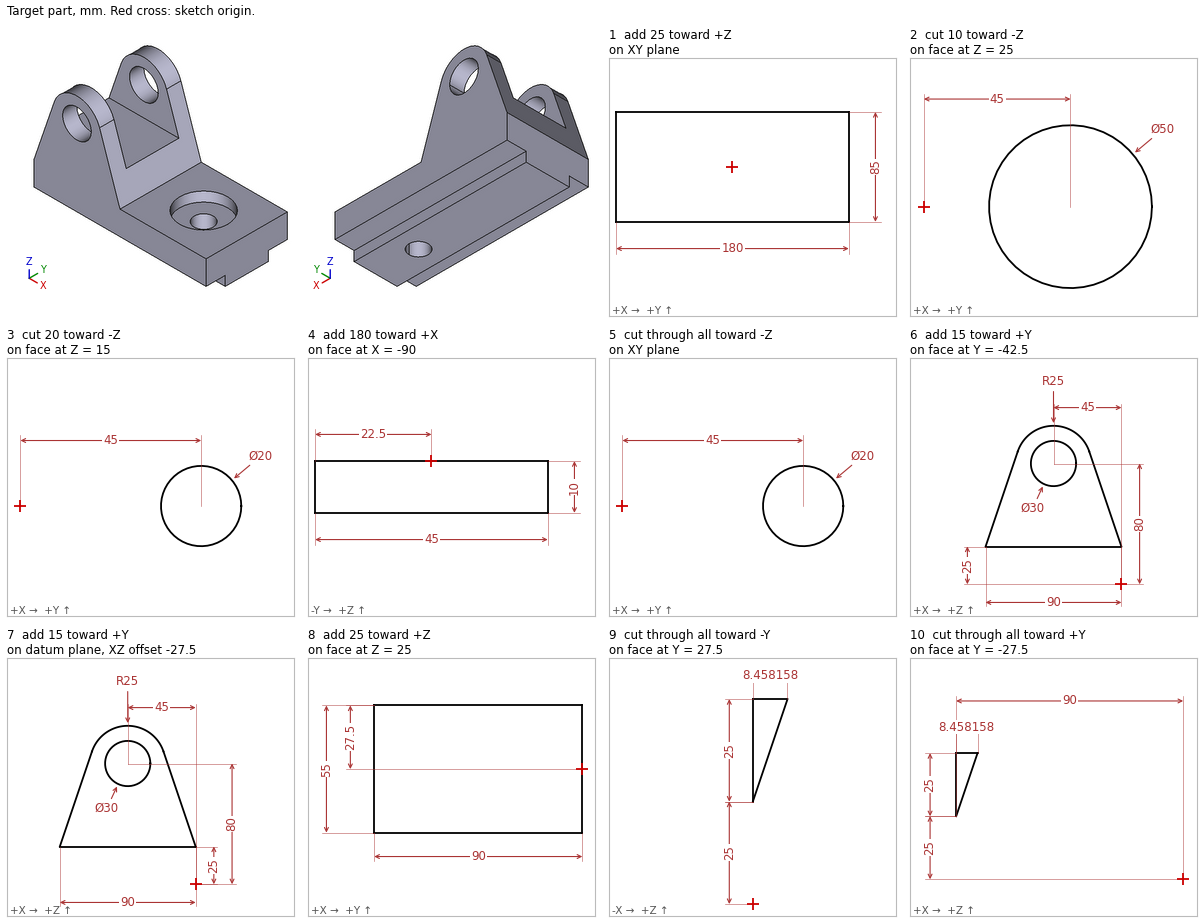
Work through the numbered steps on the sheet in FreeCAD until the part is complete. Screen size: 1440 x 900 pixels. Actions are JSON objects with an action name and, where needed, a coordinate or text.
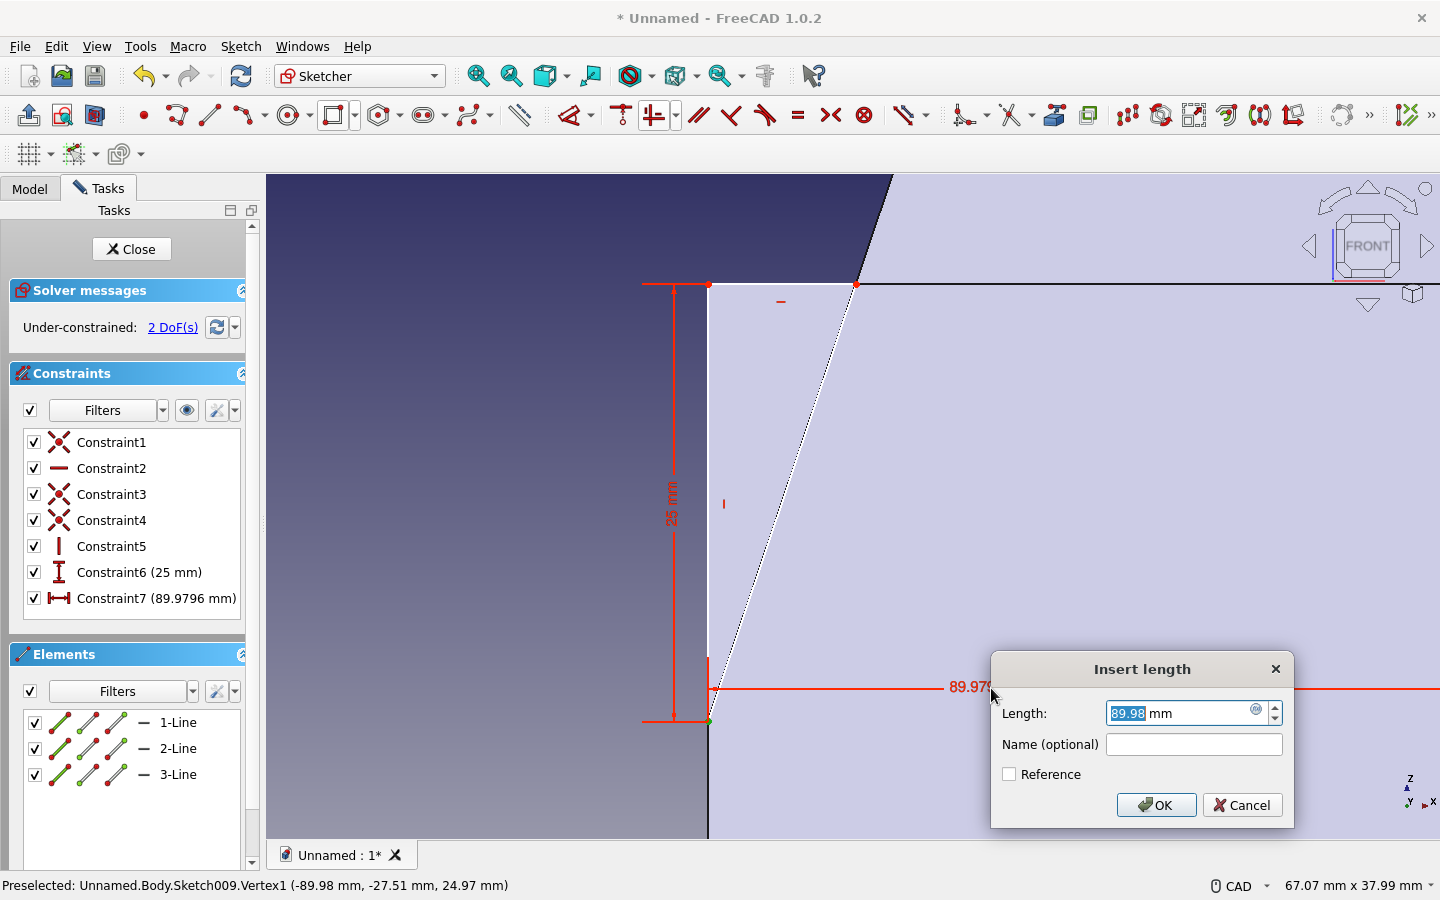
{"action": "type", "text": "90"}
{"action": "key", "text": "Return"}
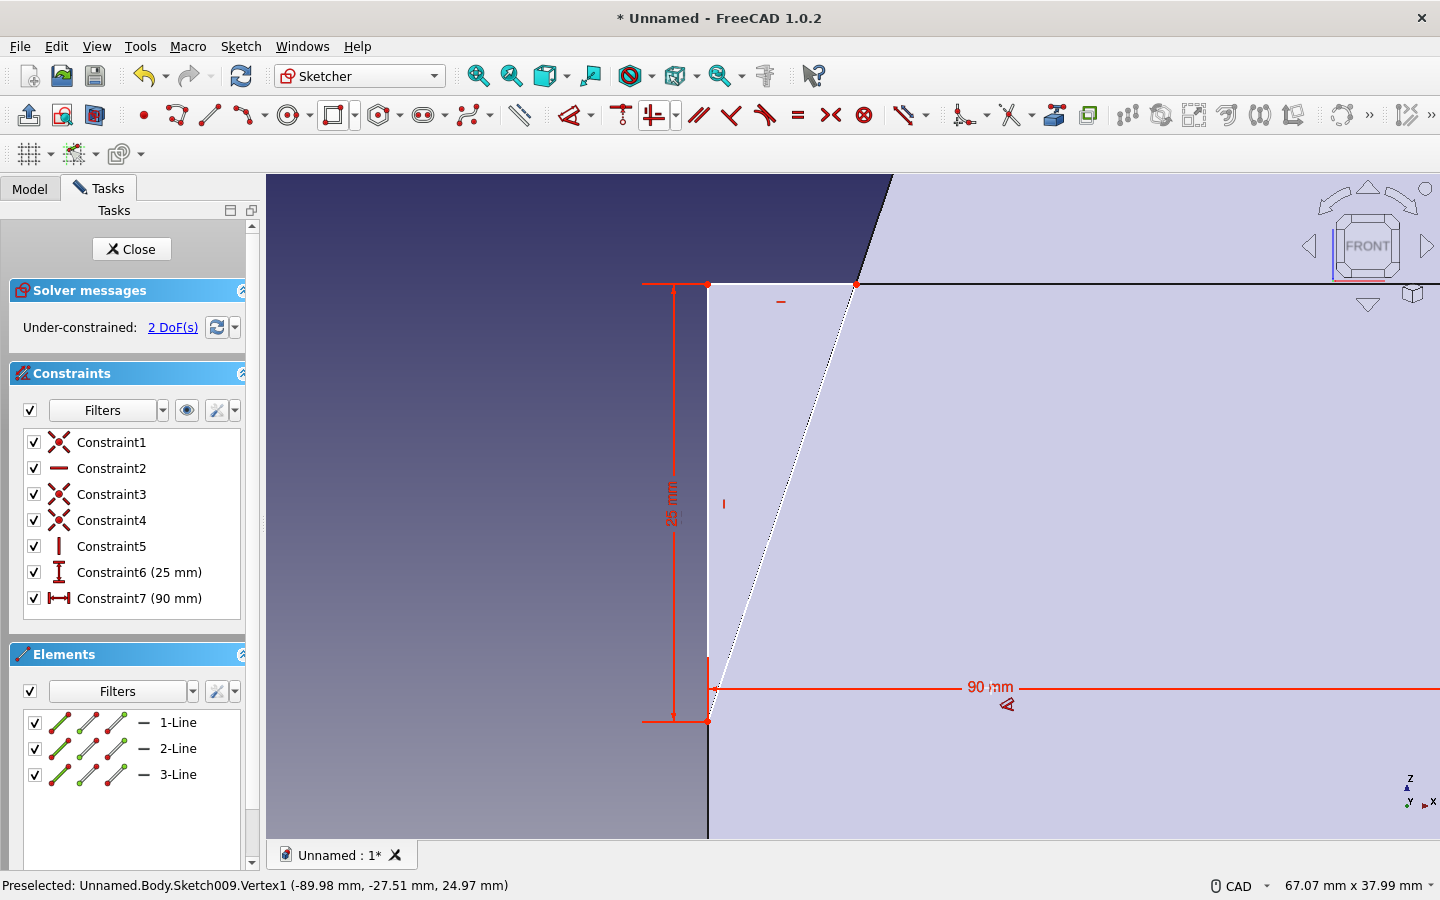
{"action": "left_click", "coordinate": [708, 722]}
{"action": "left_click", "coordinate": [674, 767]}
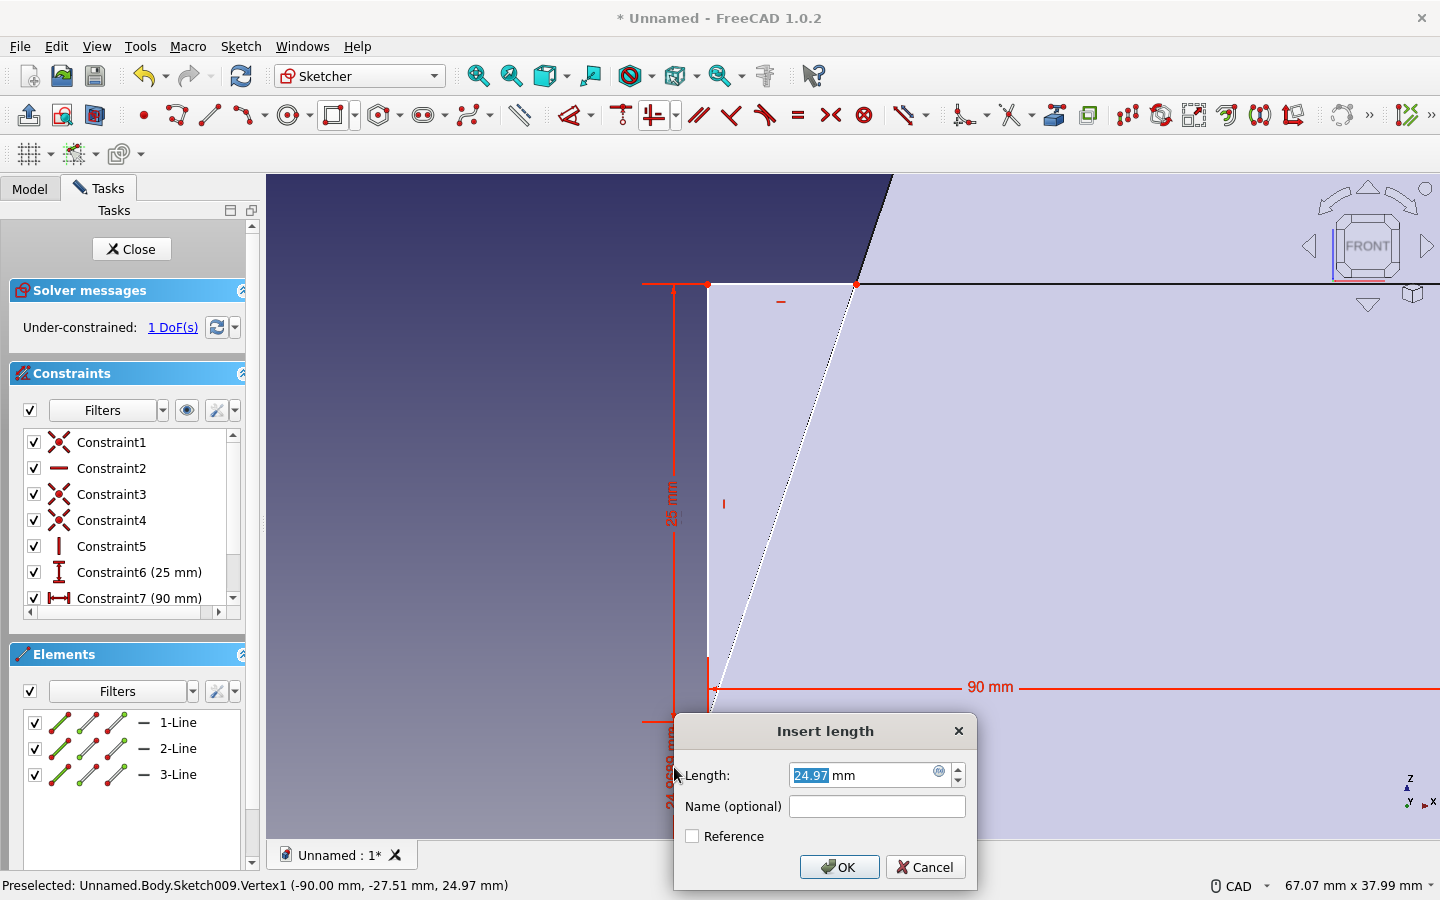
{"action": "type", "text": "25"}
{"action": "key", "text": "Return"}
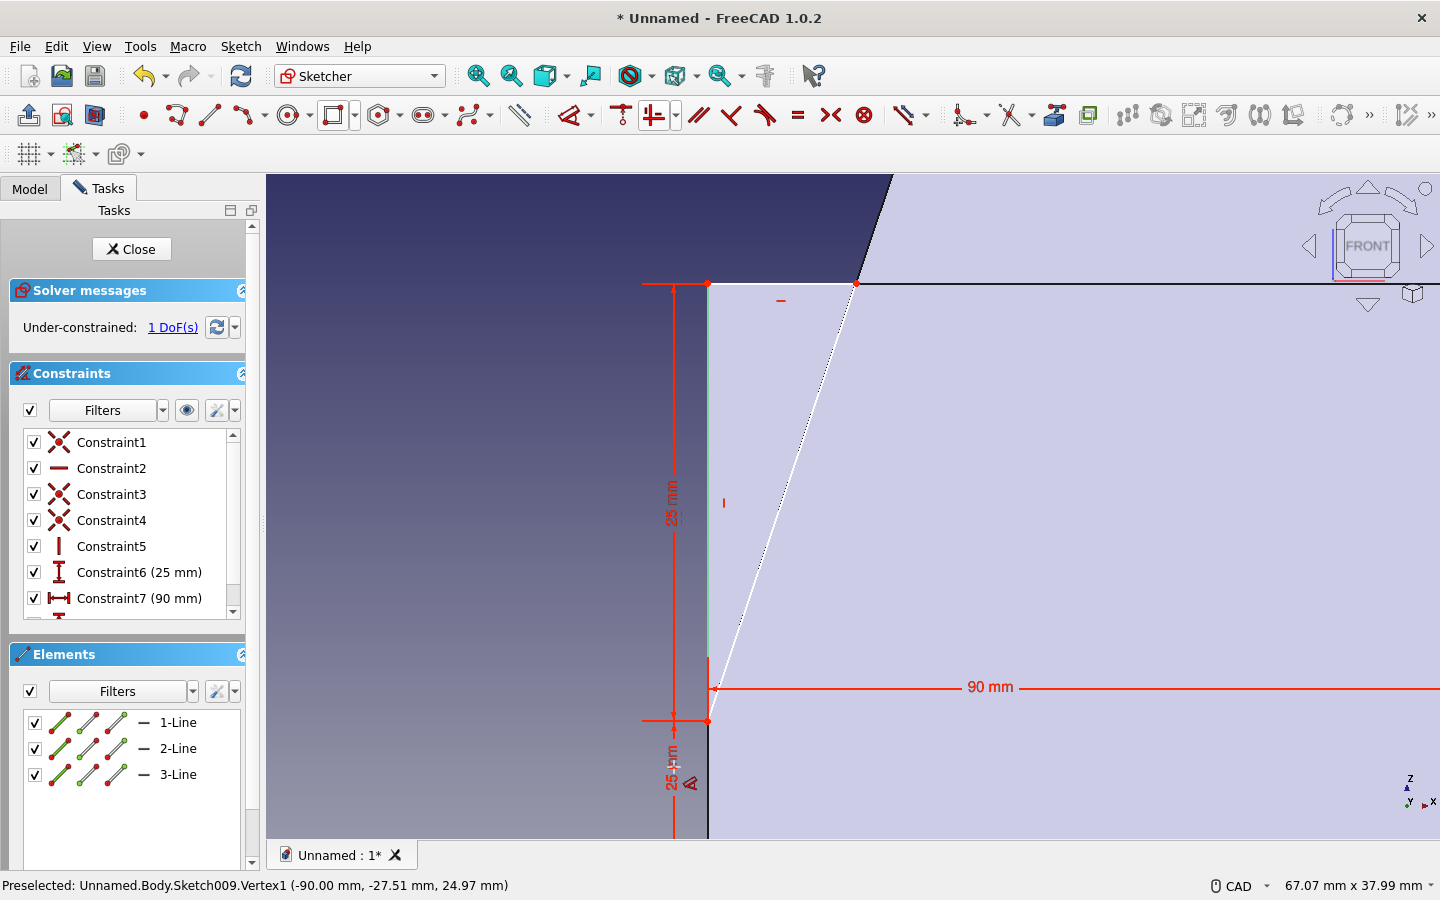
{"action": "left_click", "coordinate": [811, 284]}
{"action": "left_click", "coordinate": [782, 250]}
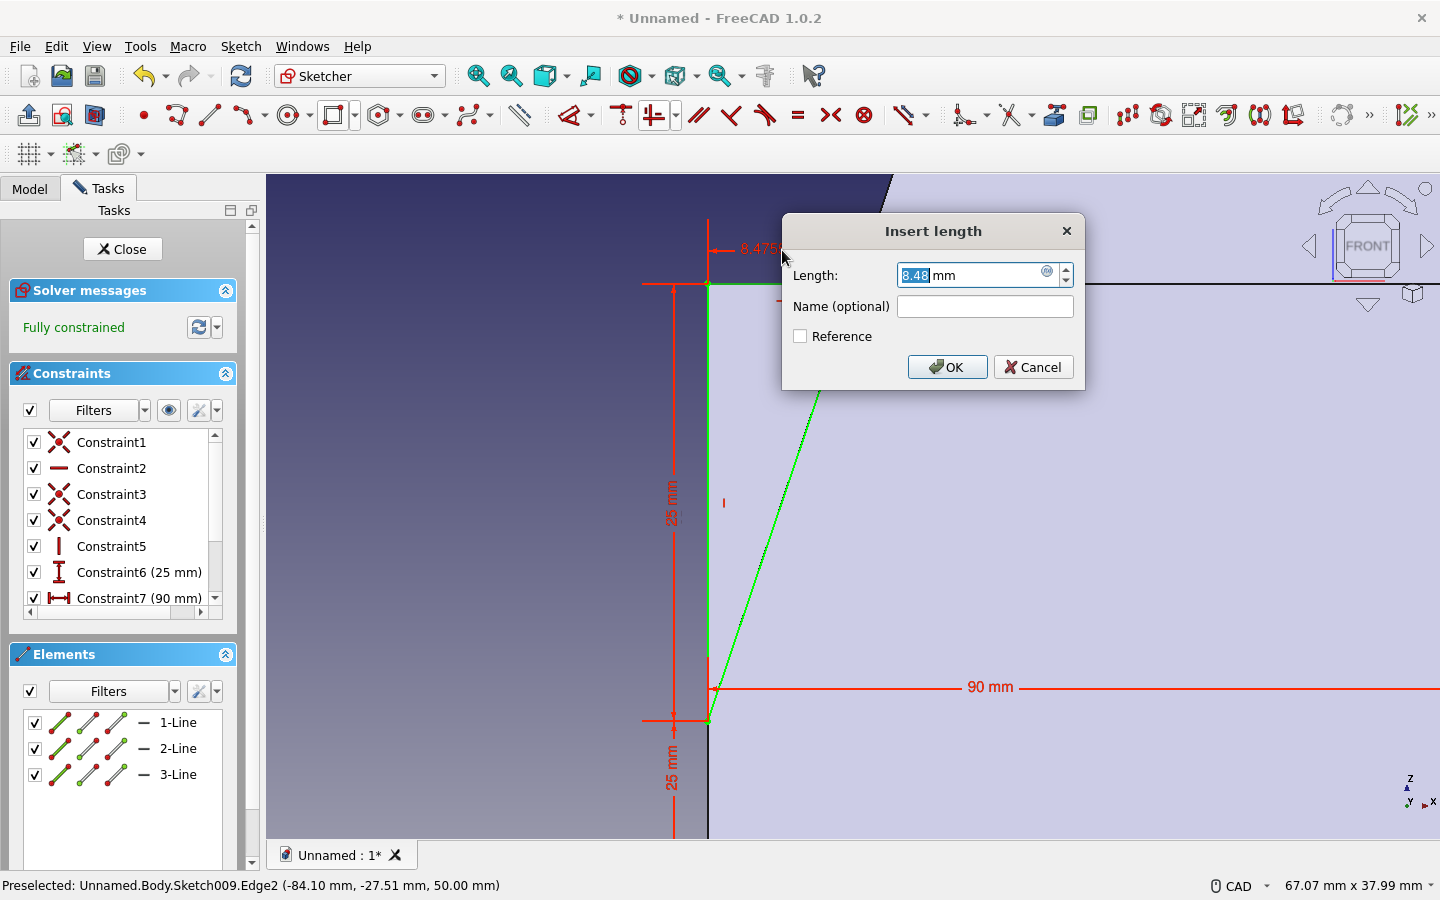
{"action": "type", "text": "8.458158"}
{"action": "key", "text": "Return"}
{"action": "key", "text": "Escape"}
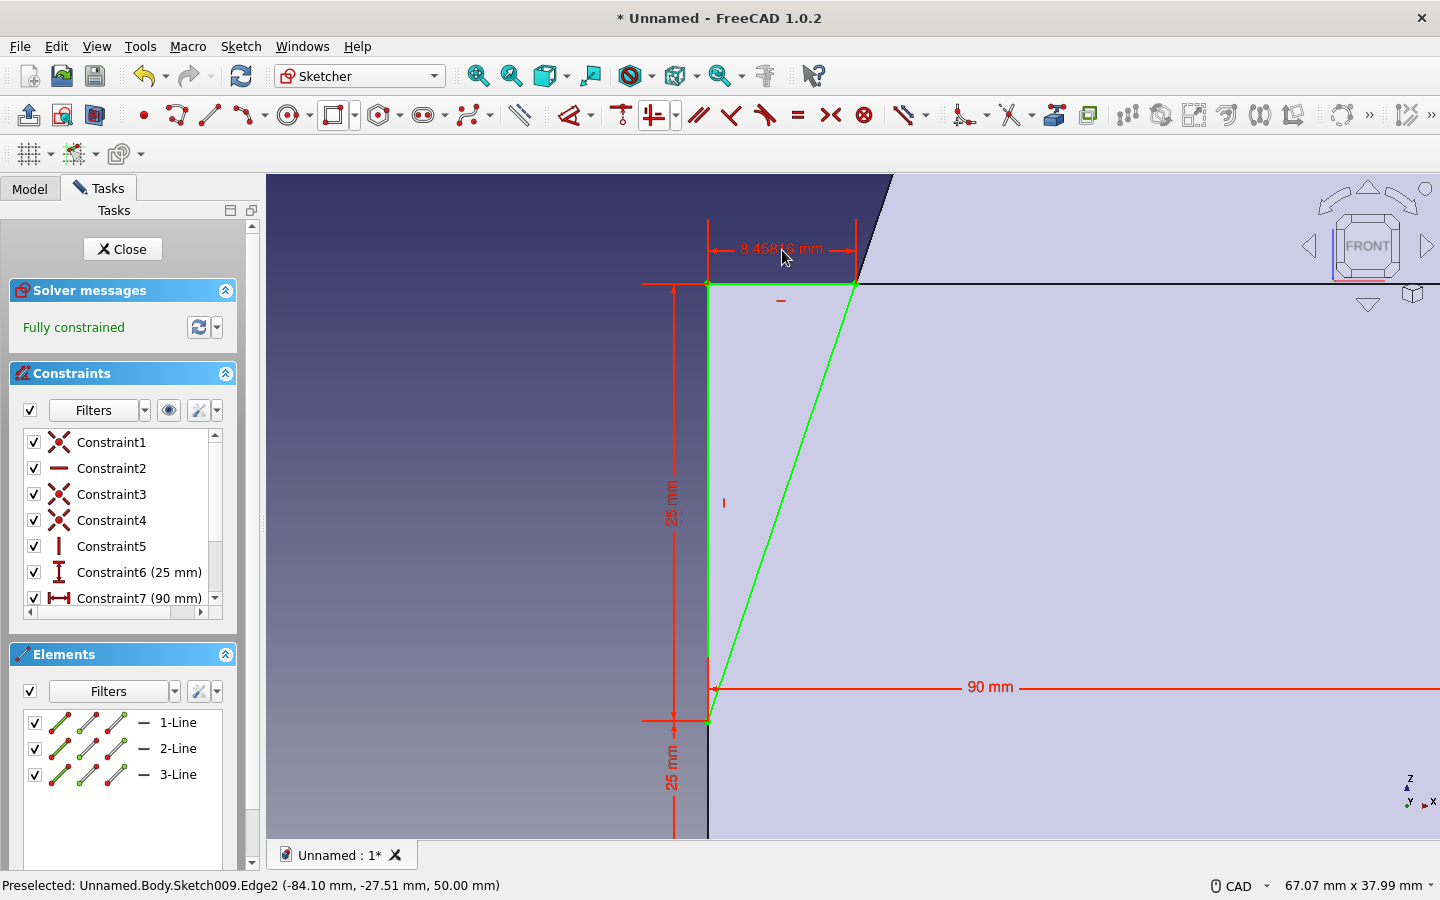
{"action": "left_click", "coordinate": [123, 249]}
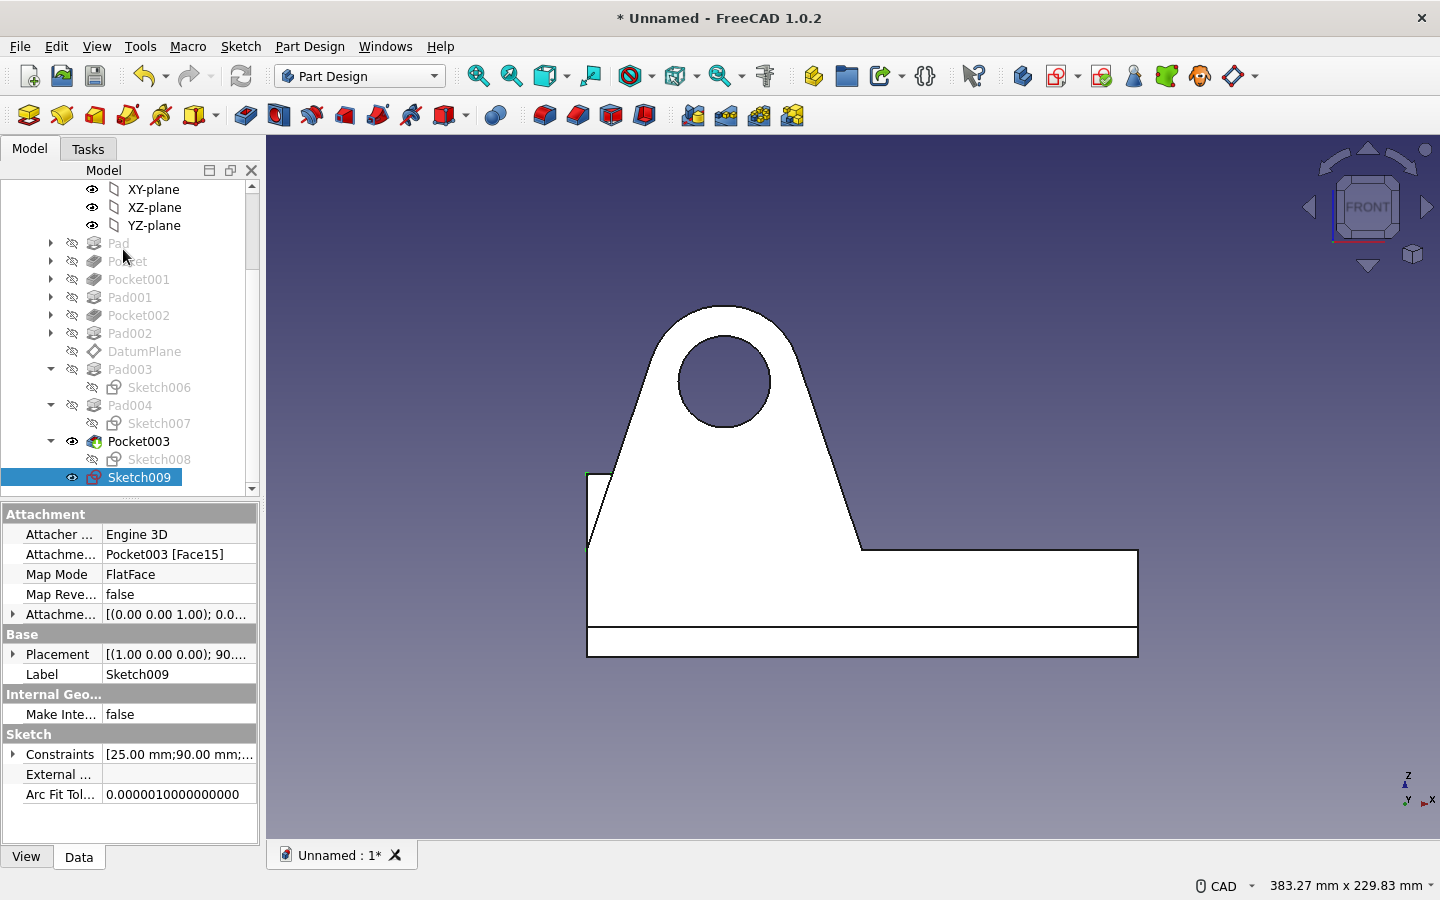
{"action": "left_click", "coordinate": [246, 116]}